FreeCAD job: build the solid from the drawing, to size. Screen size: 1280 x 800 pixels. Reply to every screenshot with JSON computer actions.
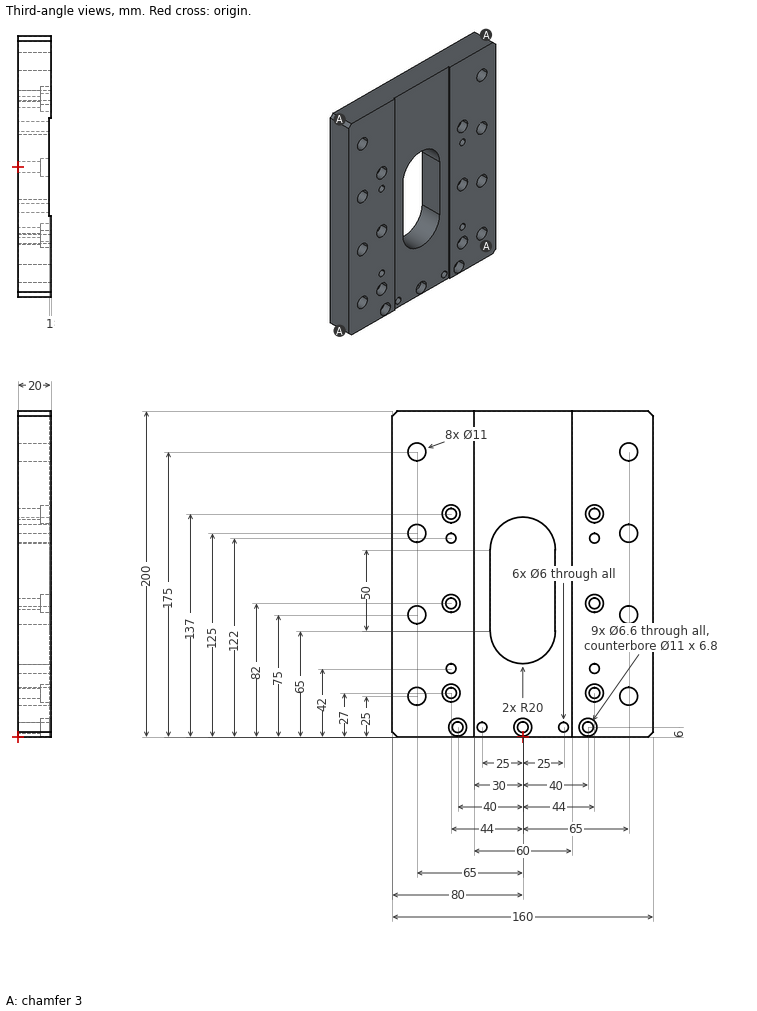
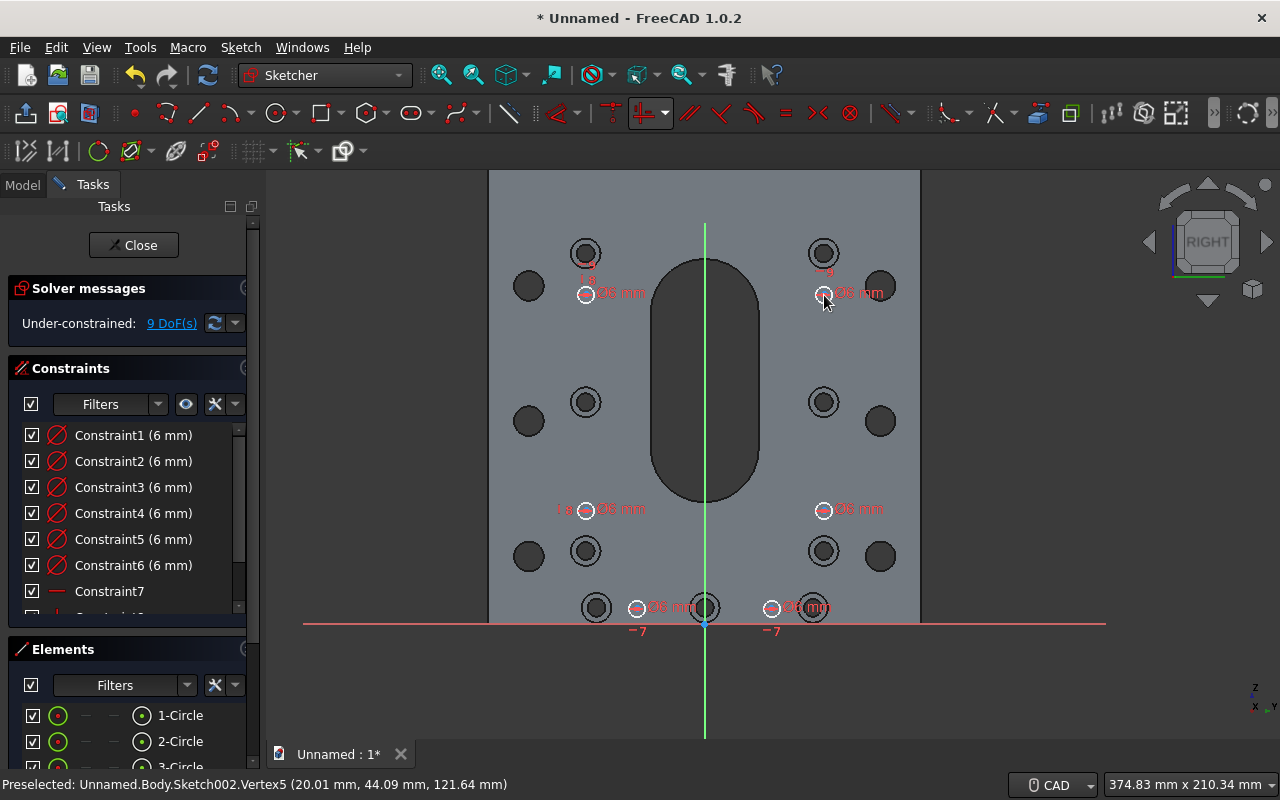
{"action": "left_click", "coordinate": [824, 295]}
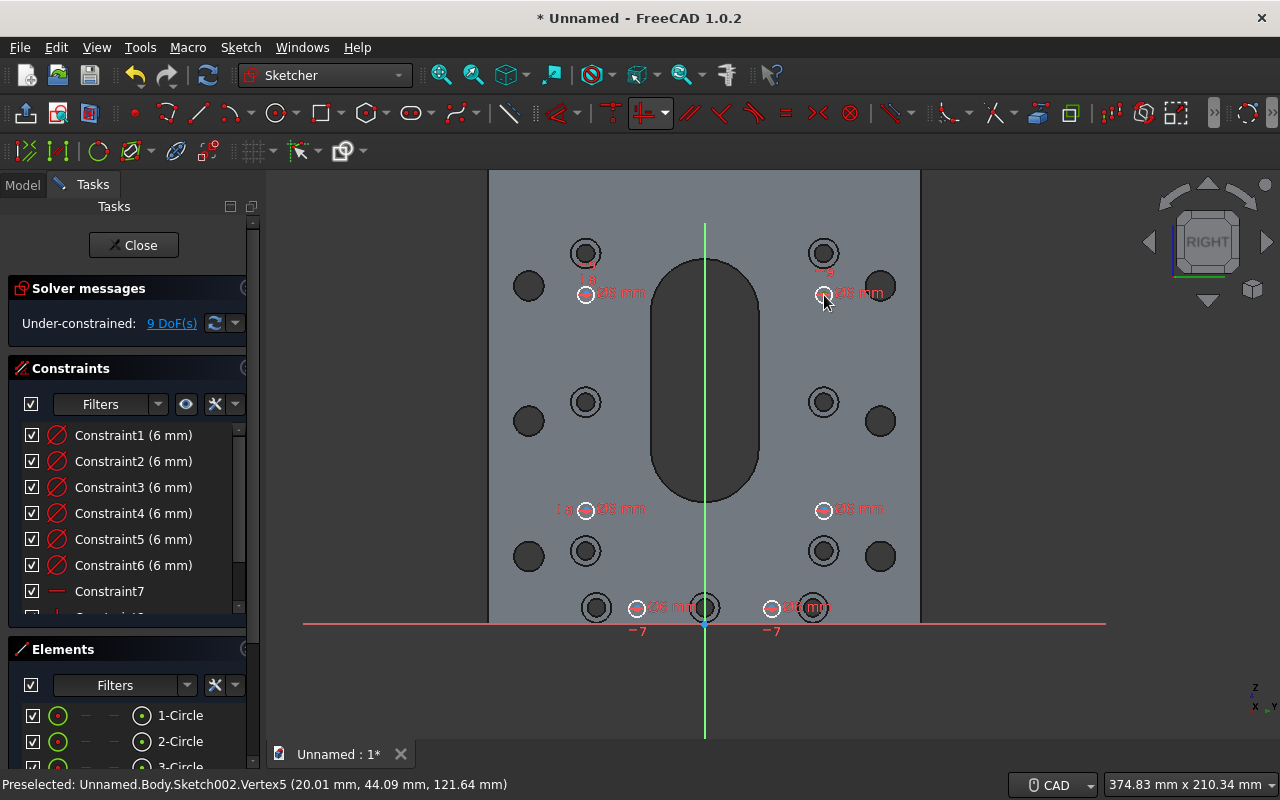
{"action": "left_click", "coordinate": [824, 511]}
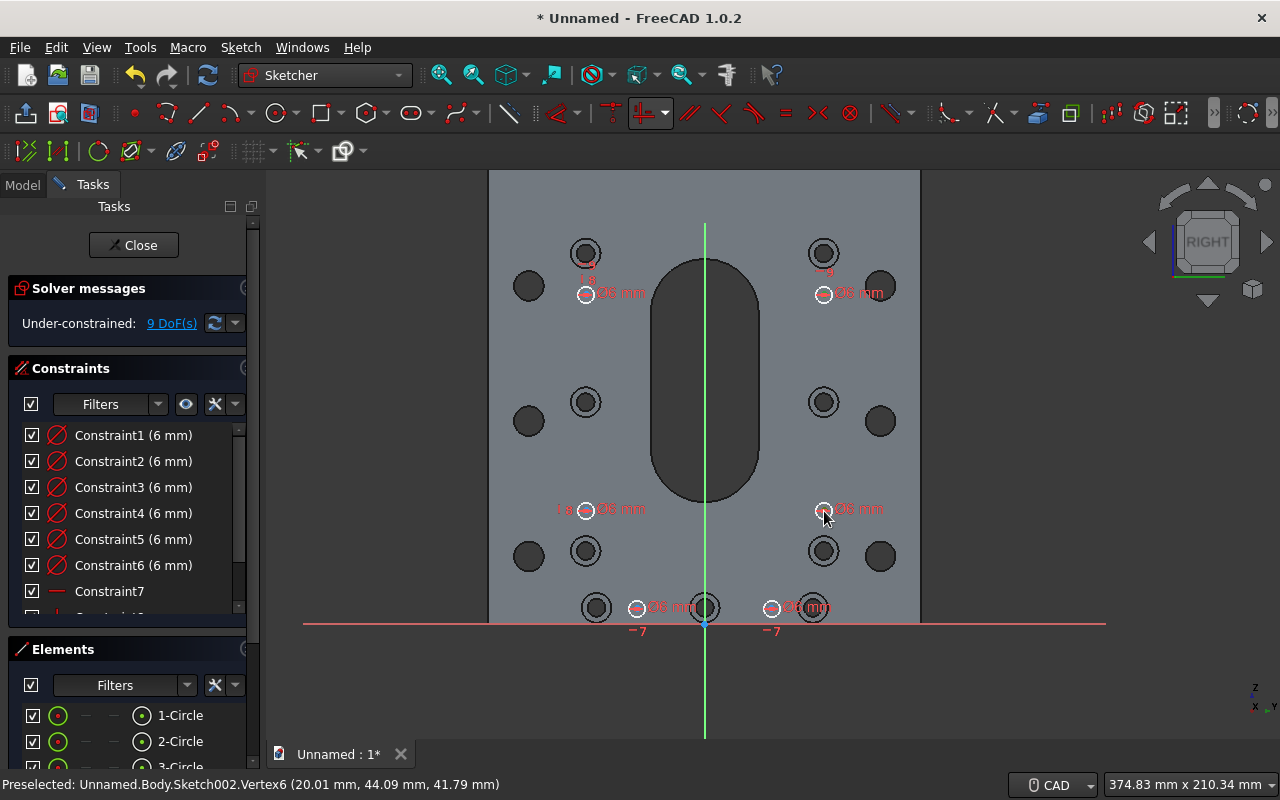
{"action": "key", "text": "v"}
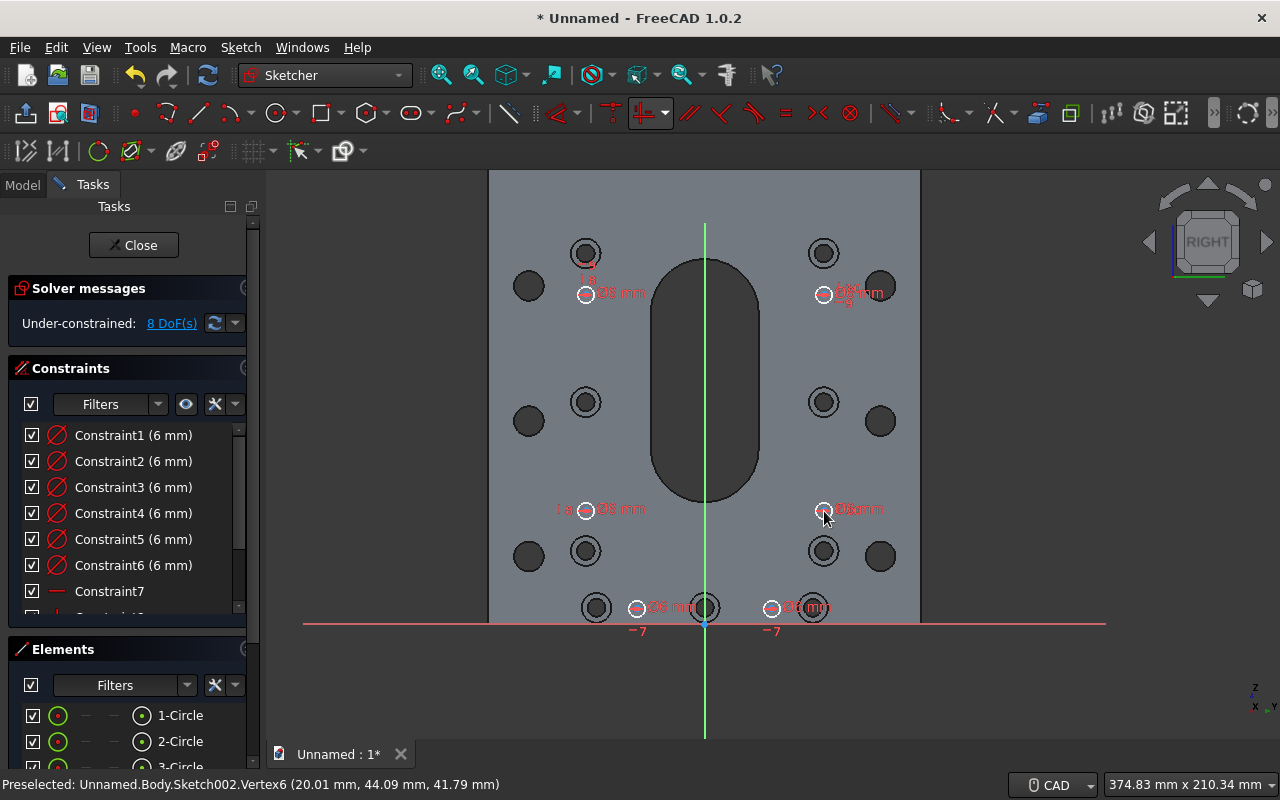
{"action": "left_click", "coordinate": [586, 511]}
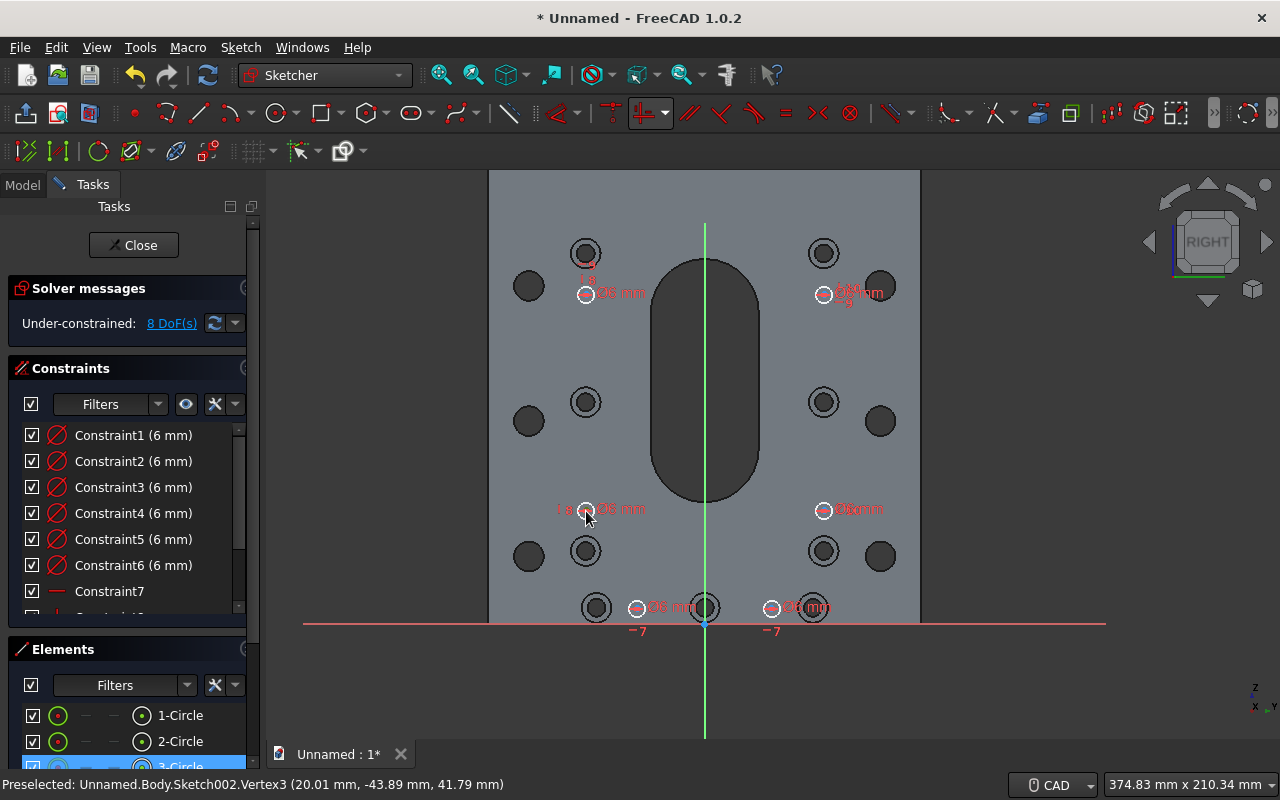
{"action": "left_click", "coordinate": [824, 511]}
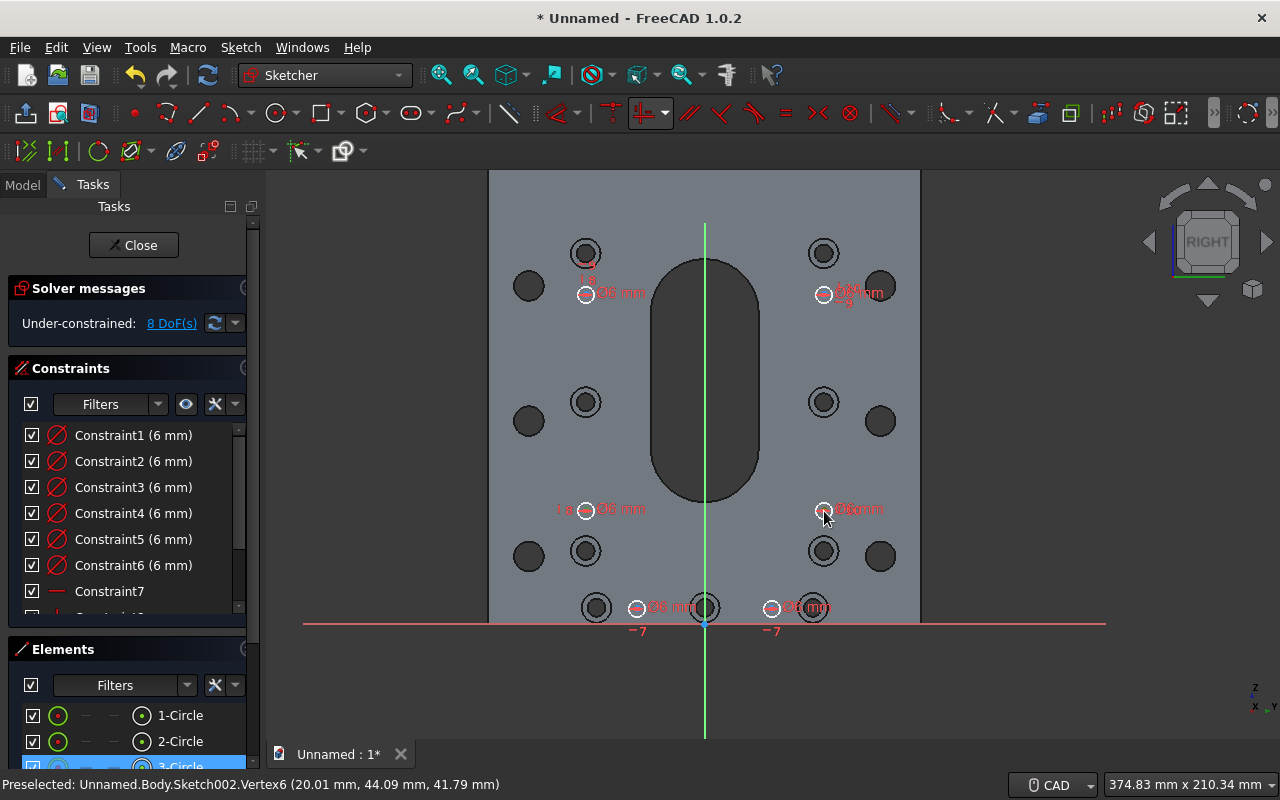
{"action": "key", "text": "h"}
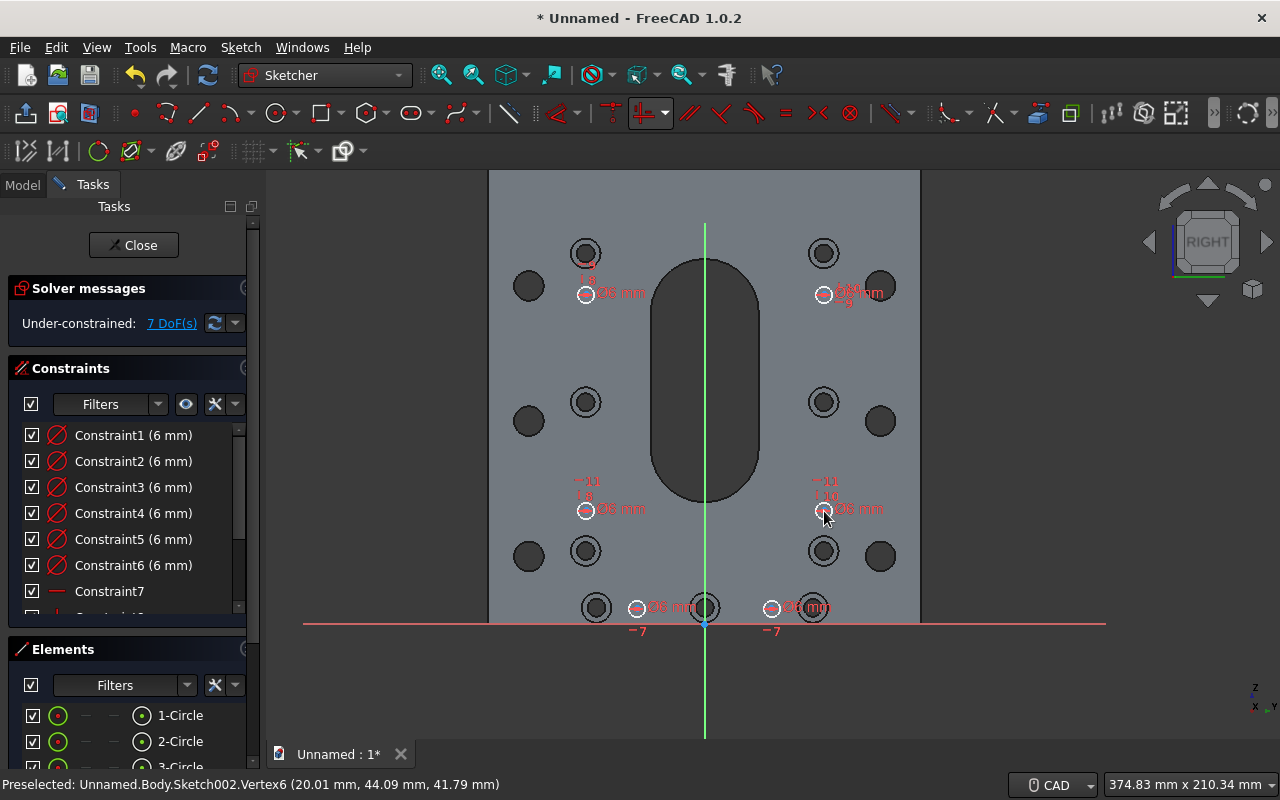
{"action": "key", "text": "d"}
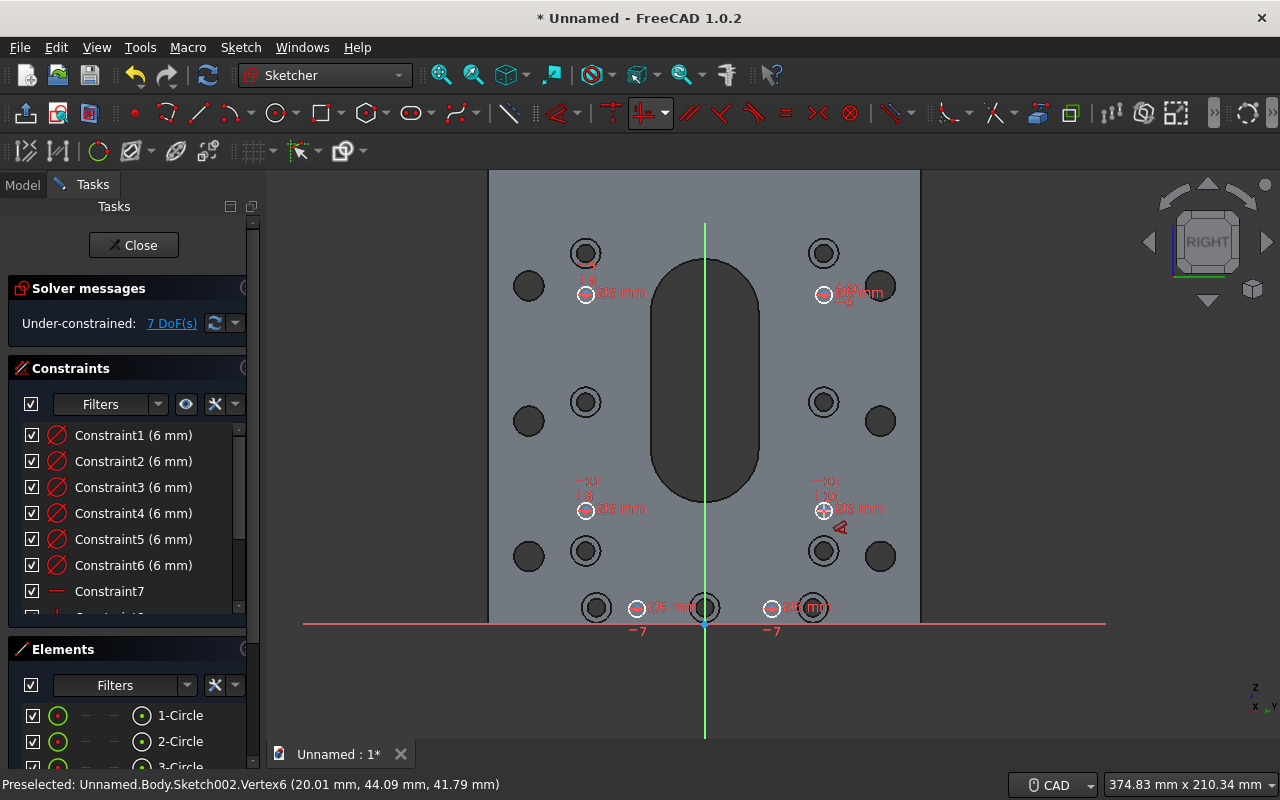
{"action": "scroll", "coordinate": [772, 609], "scroll_direction": "up", "scroll_amount": 5}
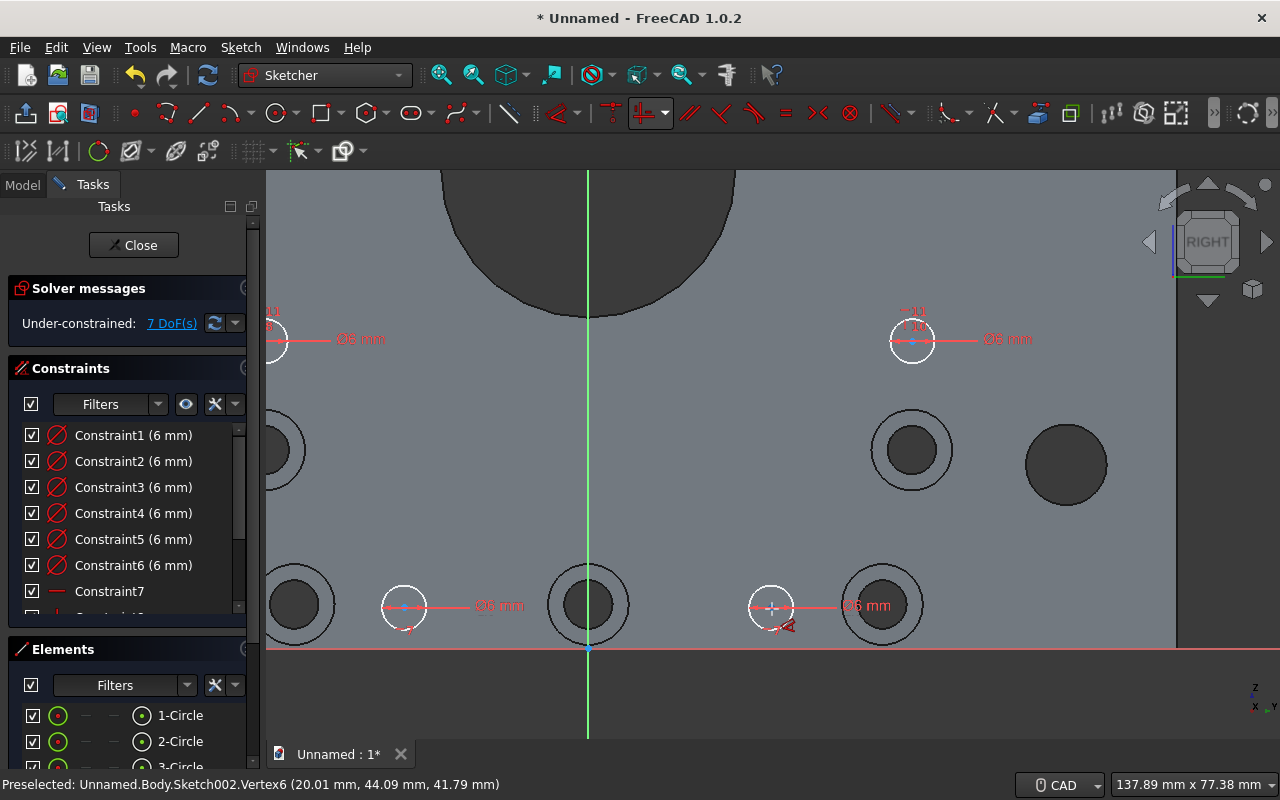
{"action": "left_click", "coordinate": [771, 608]}
{"action": "left_click", "coordinate": [805, 628]}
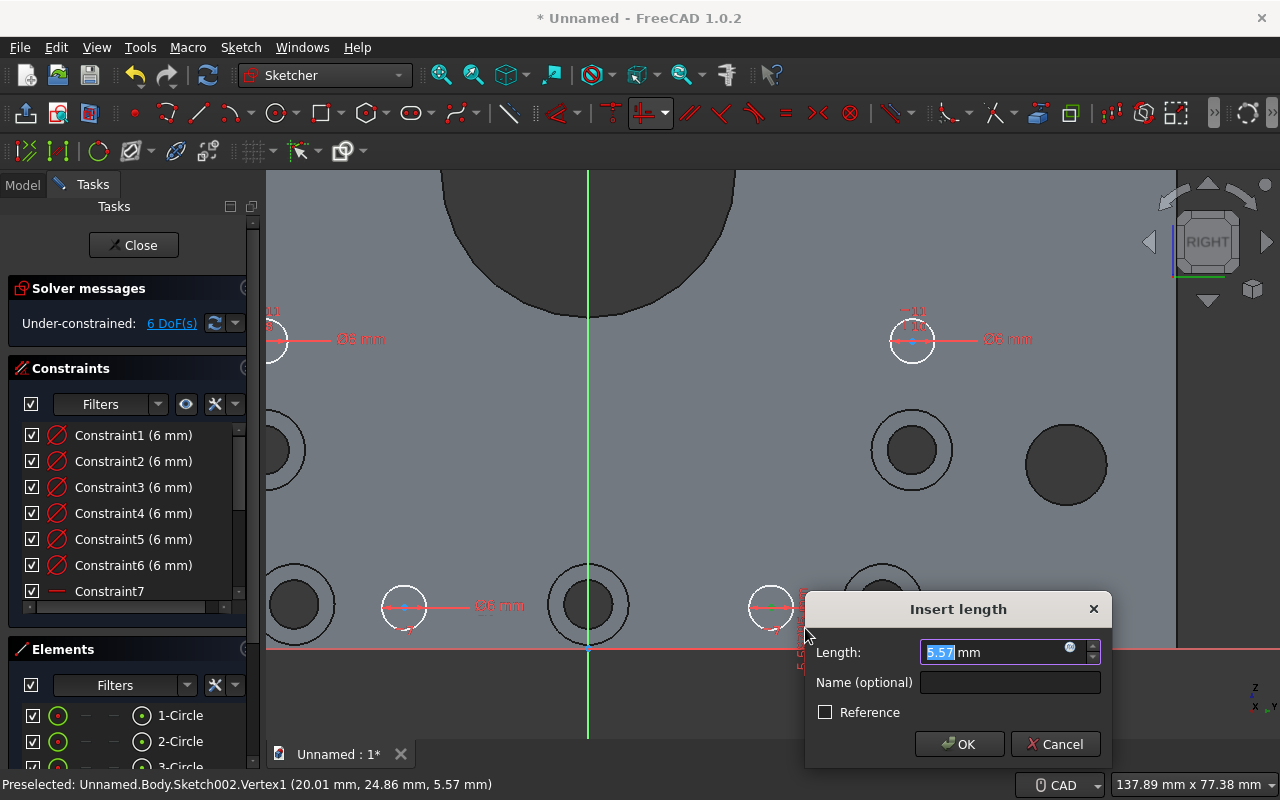
{"action": "type", "text": "6"}
{"action": "key", "text": "Return"}